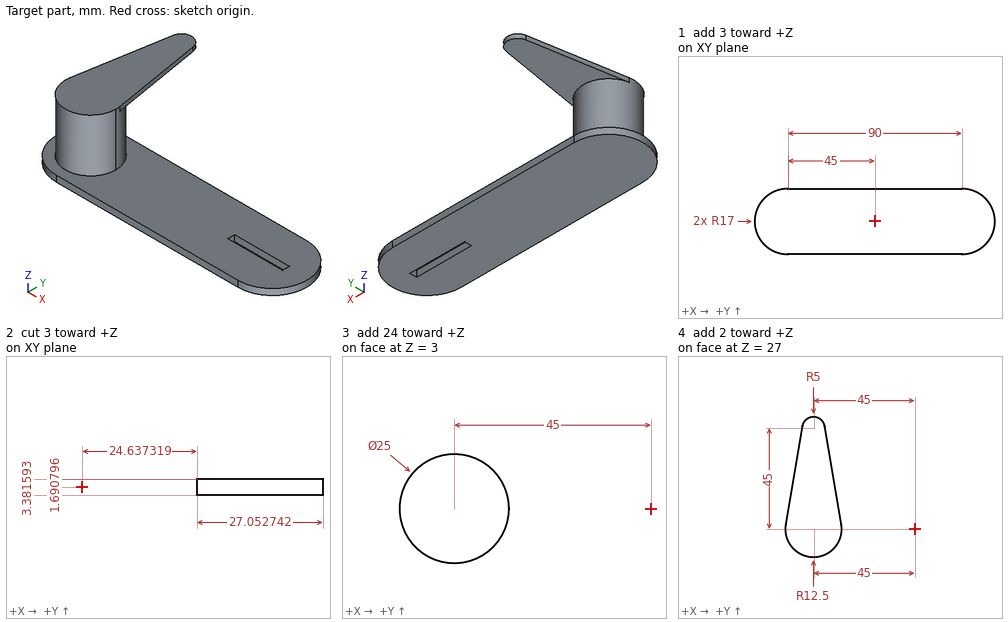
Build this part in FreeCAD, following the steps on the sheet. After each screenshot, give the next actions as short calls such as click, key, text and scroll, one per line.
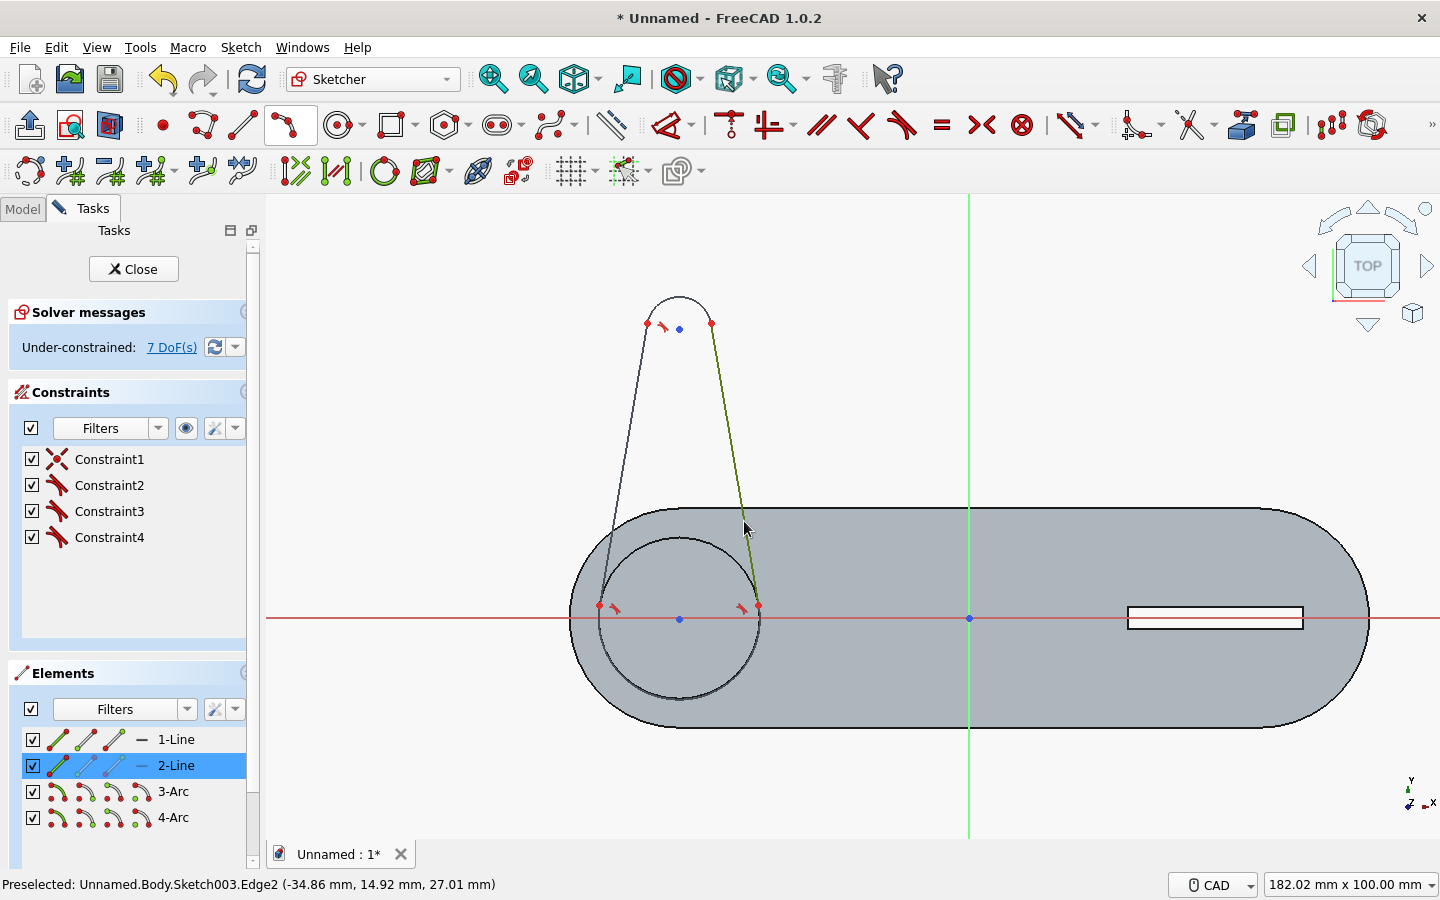
click(696, 302)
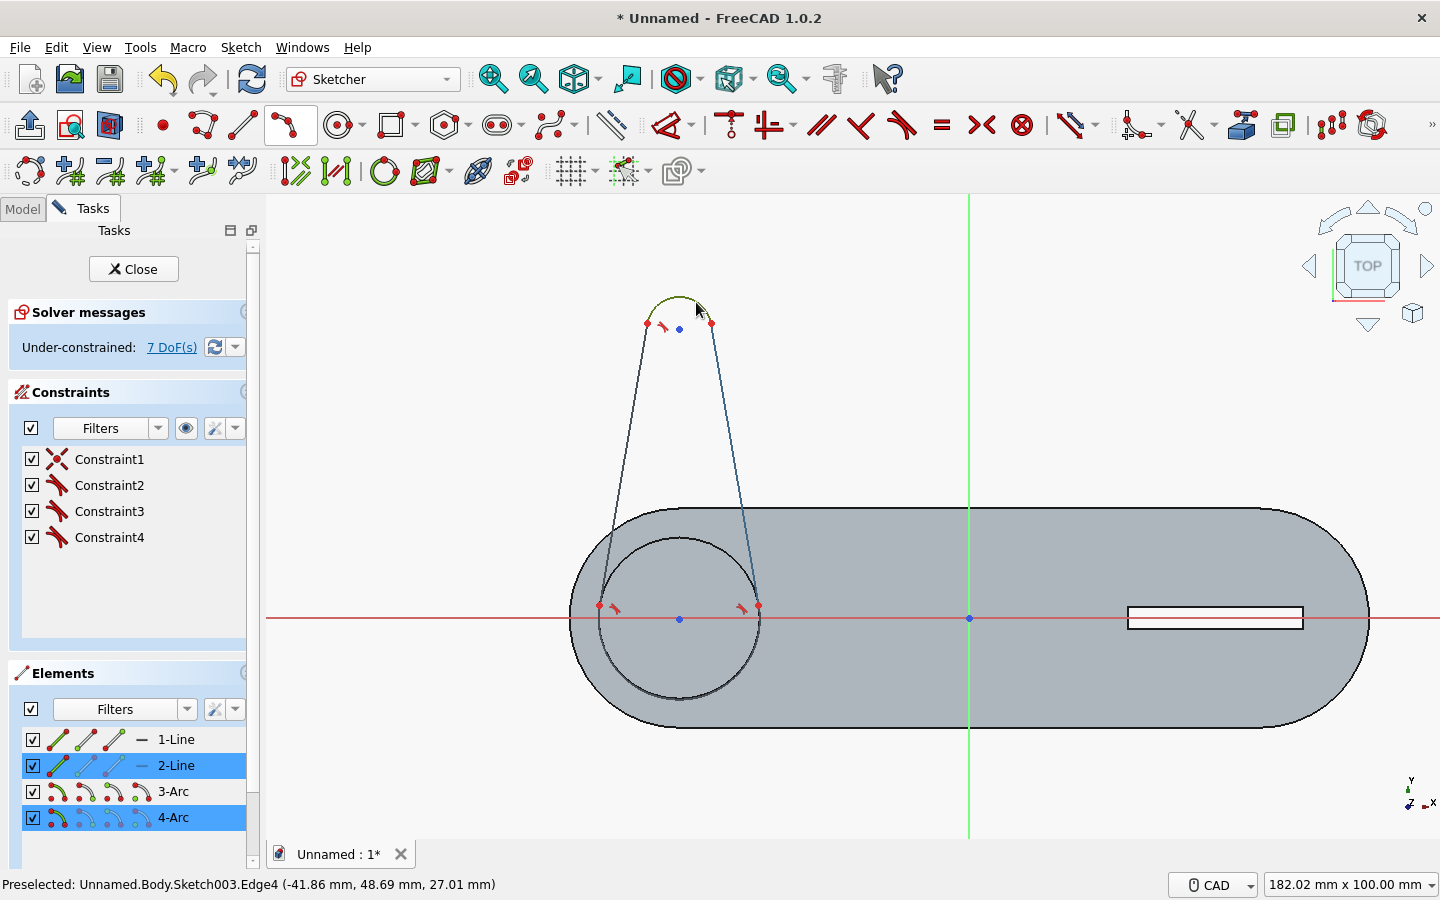
click(902, 126)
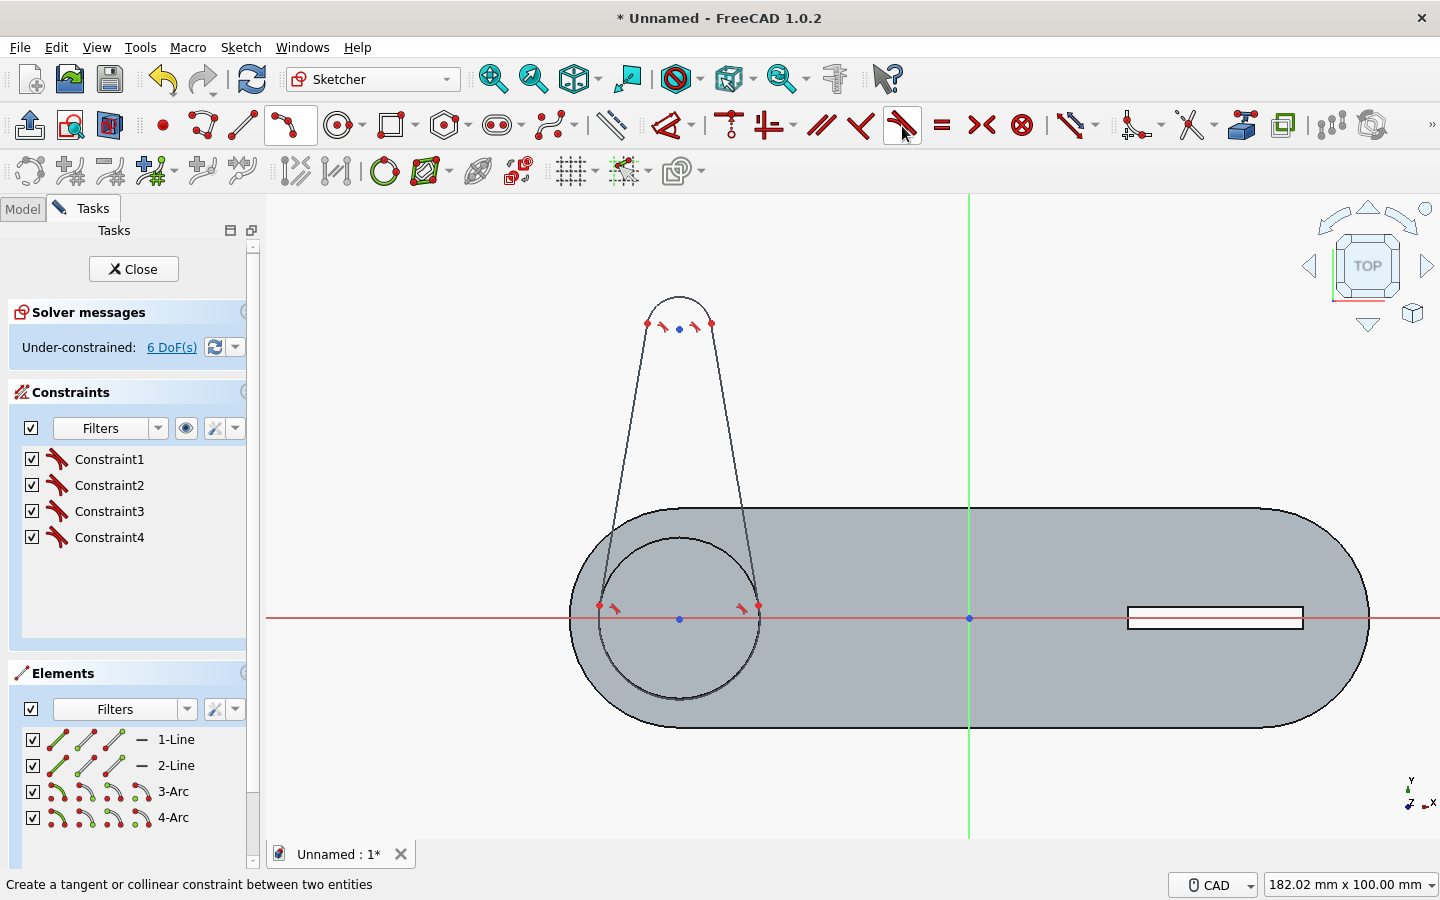
click(679, 619)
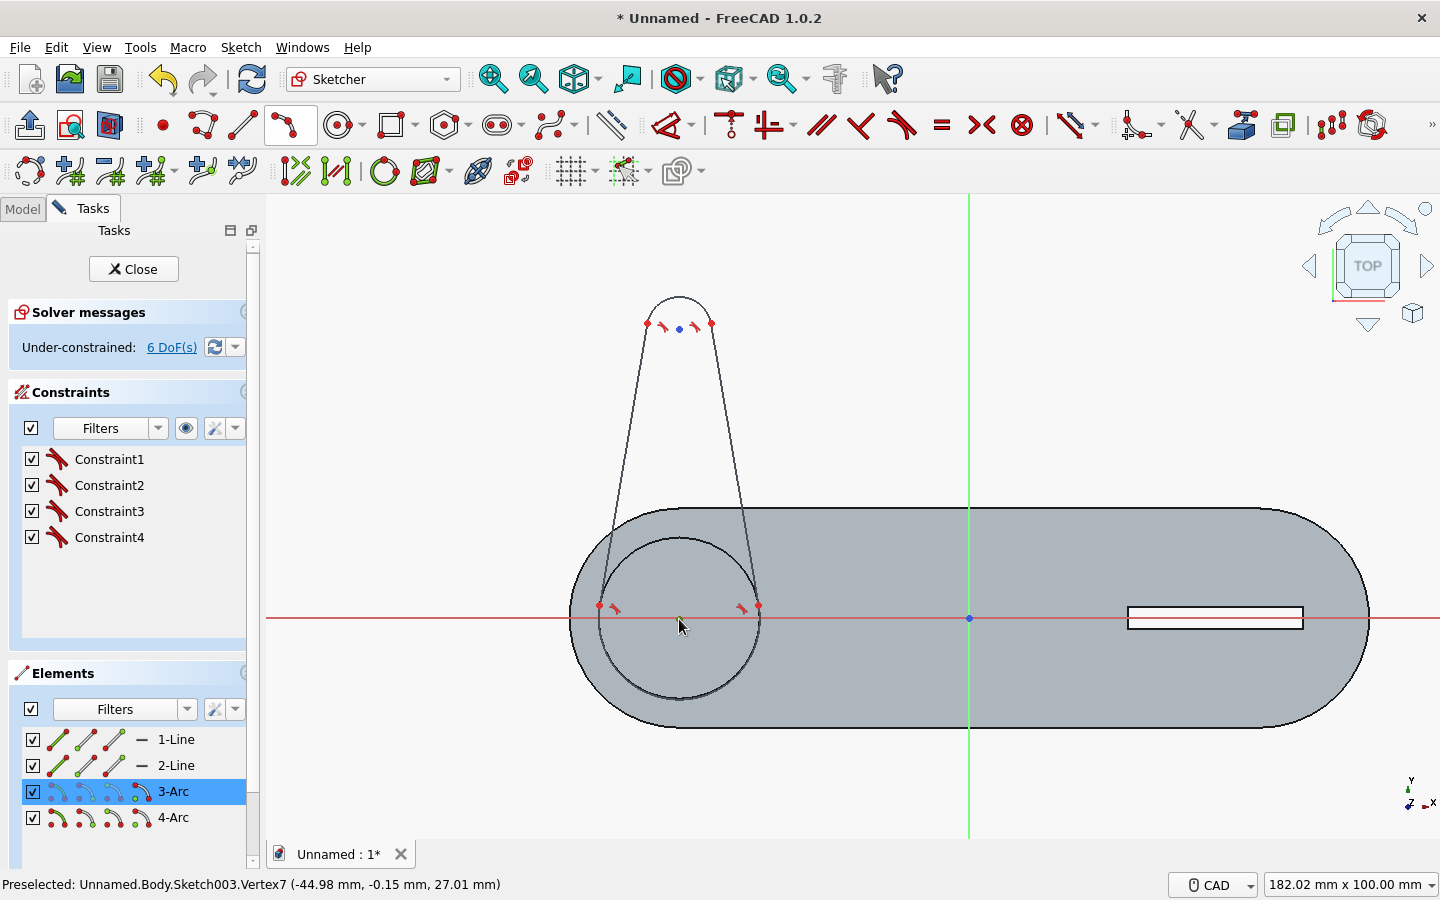
click(364, 618)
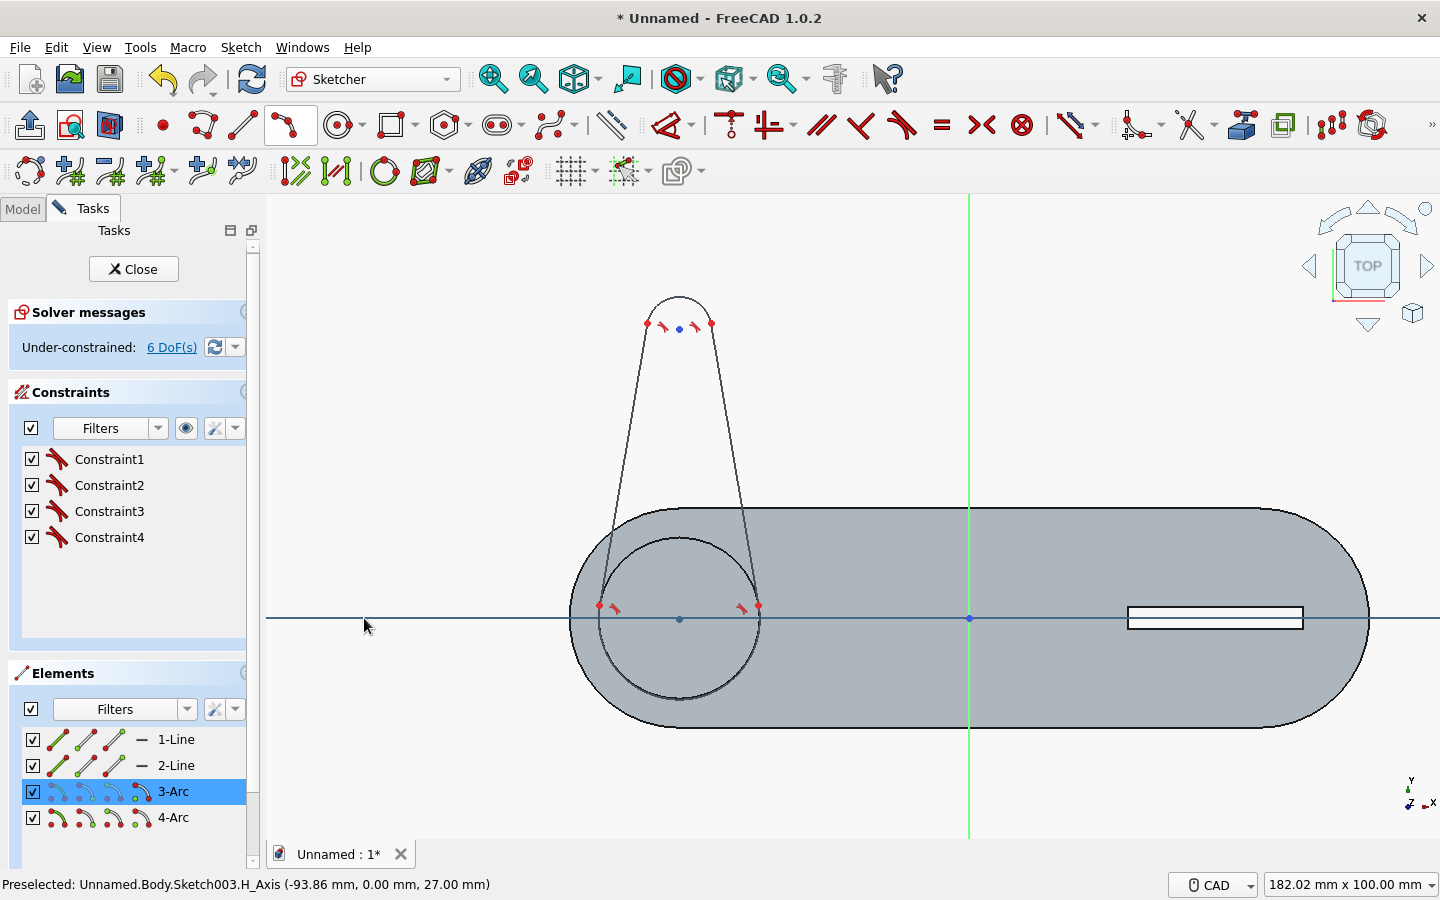
click(730, 126)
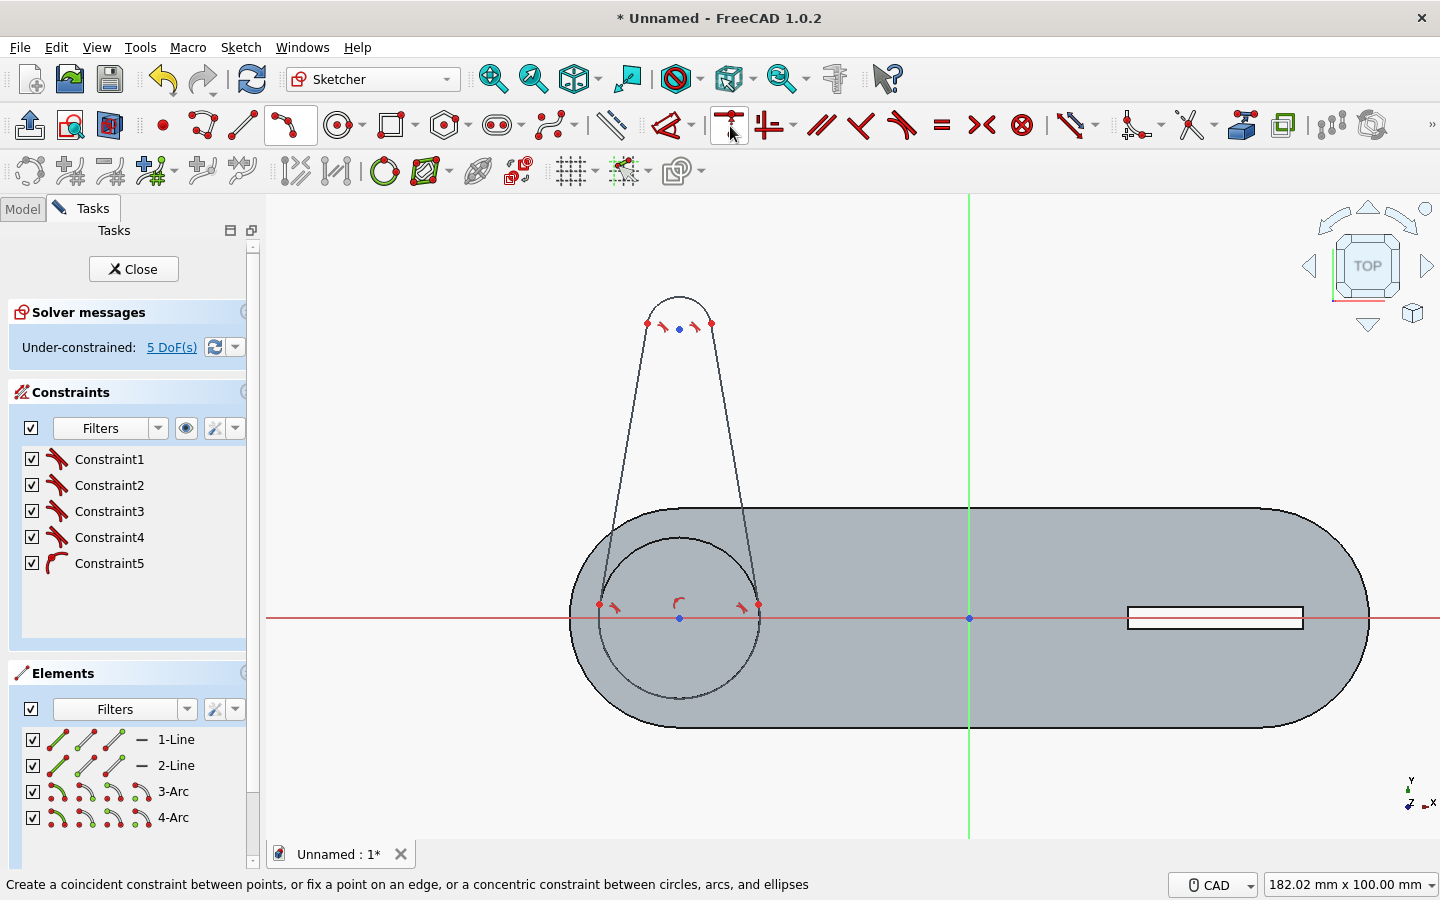
click(666, 126)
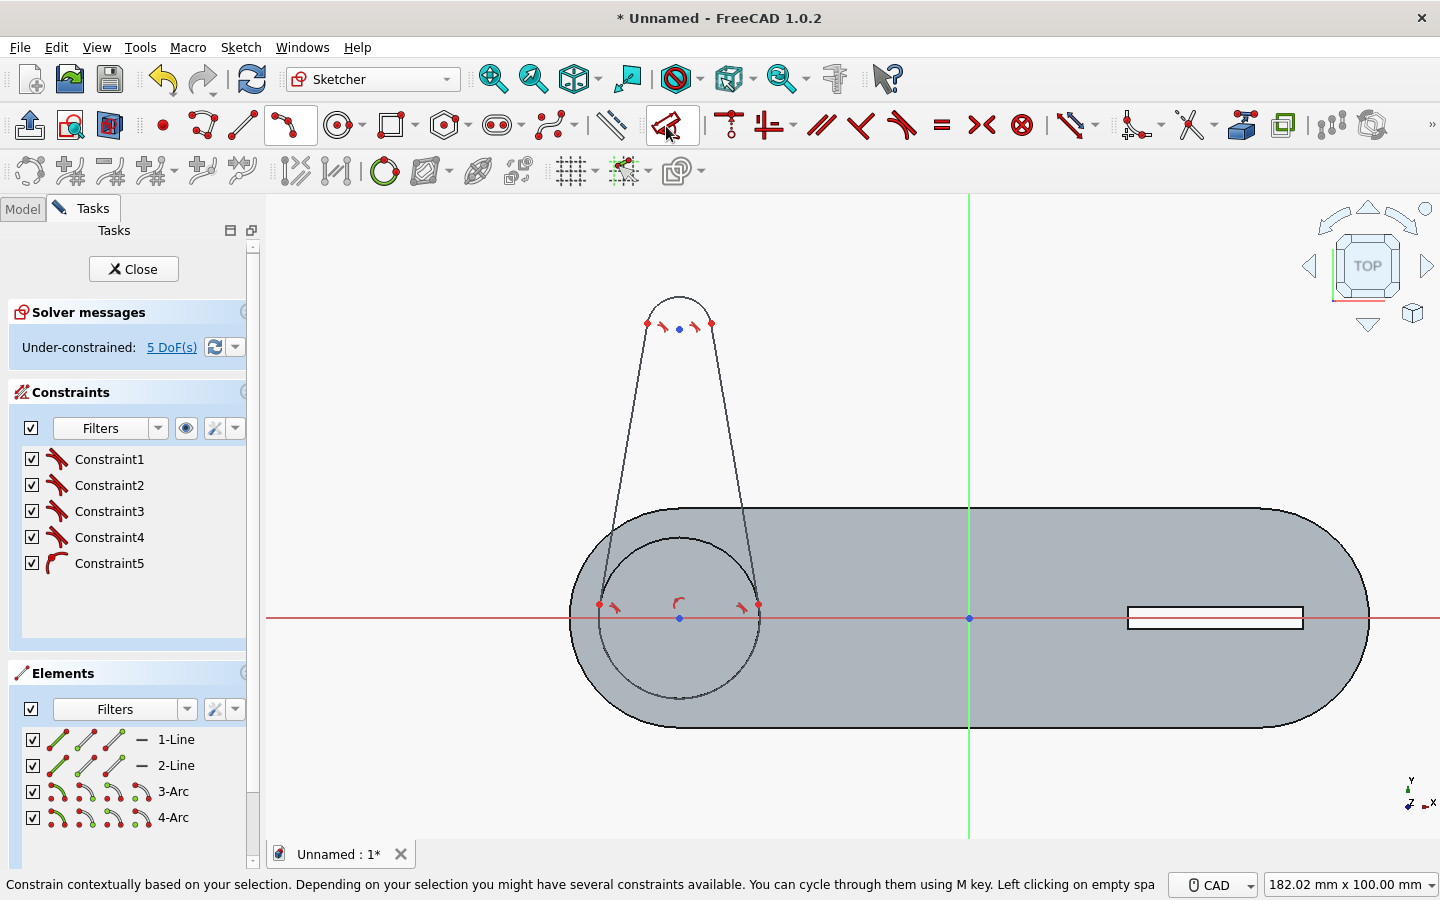
click(628, 680)
click(608, 705)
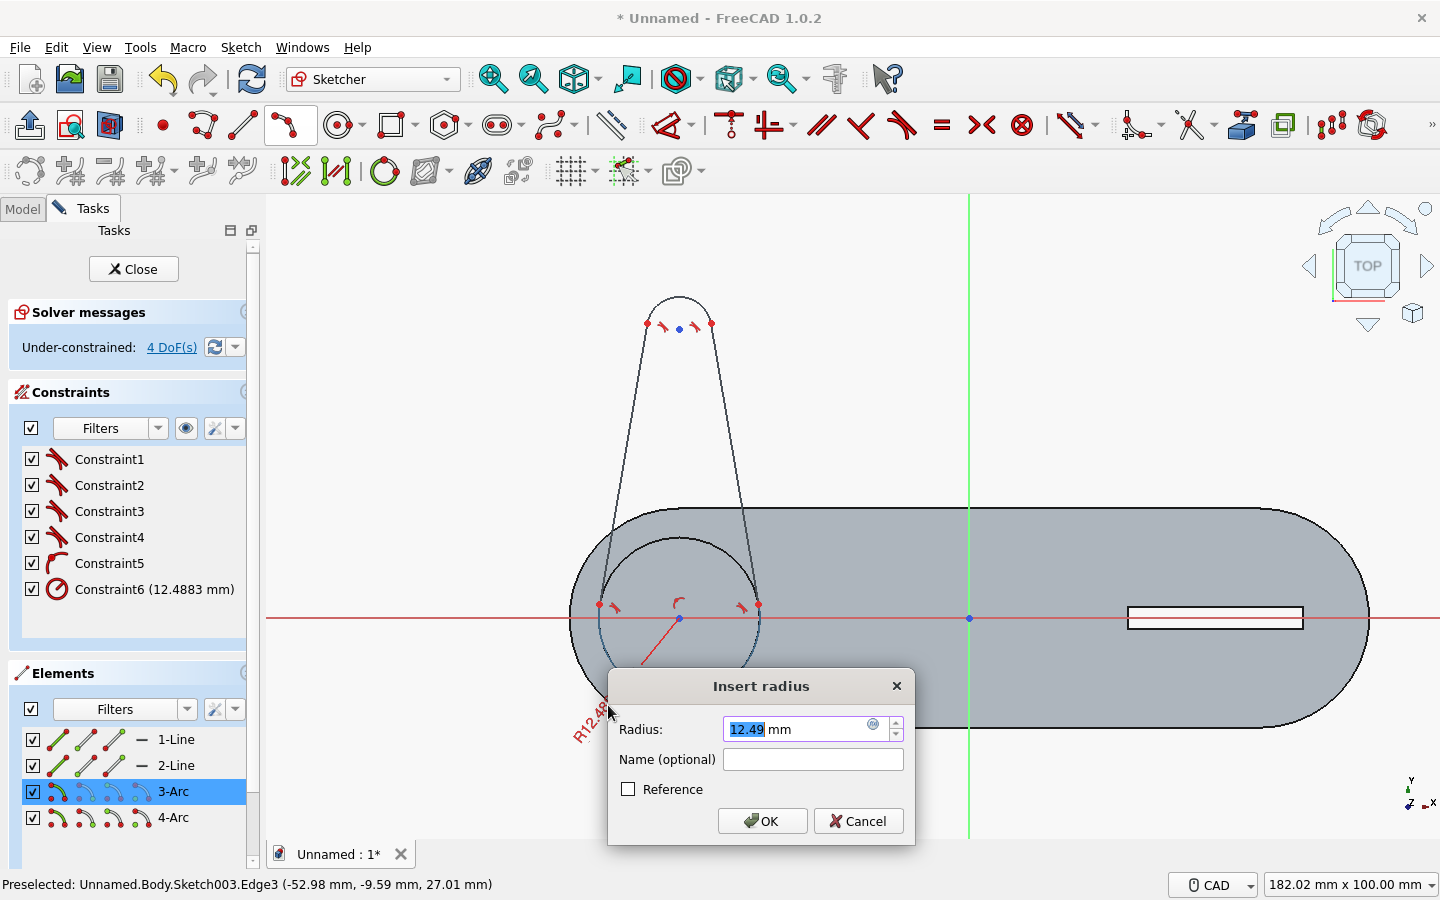
text(12.5)
key(Return)